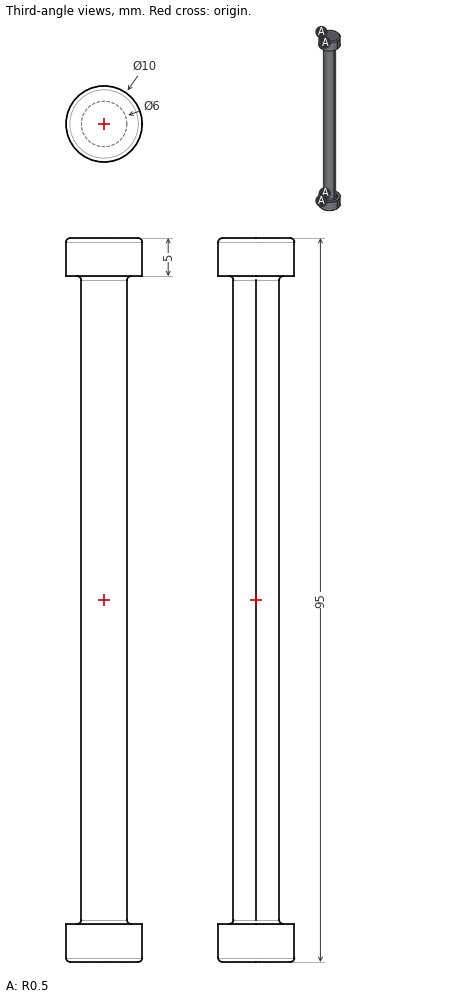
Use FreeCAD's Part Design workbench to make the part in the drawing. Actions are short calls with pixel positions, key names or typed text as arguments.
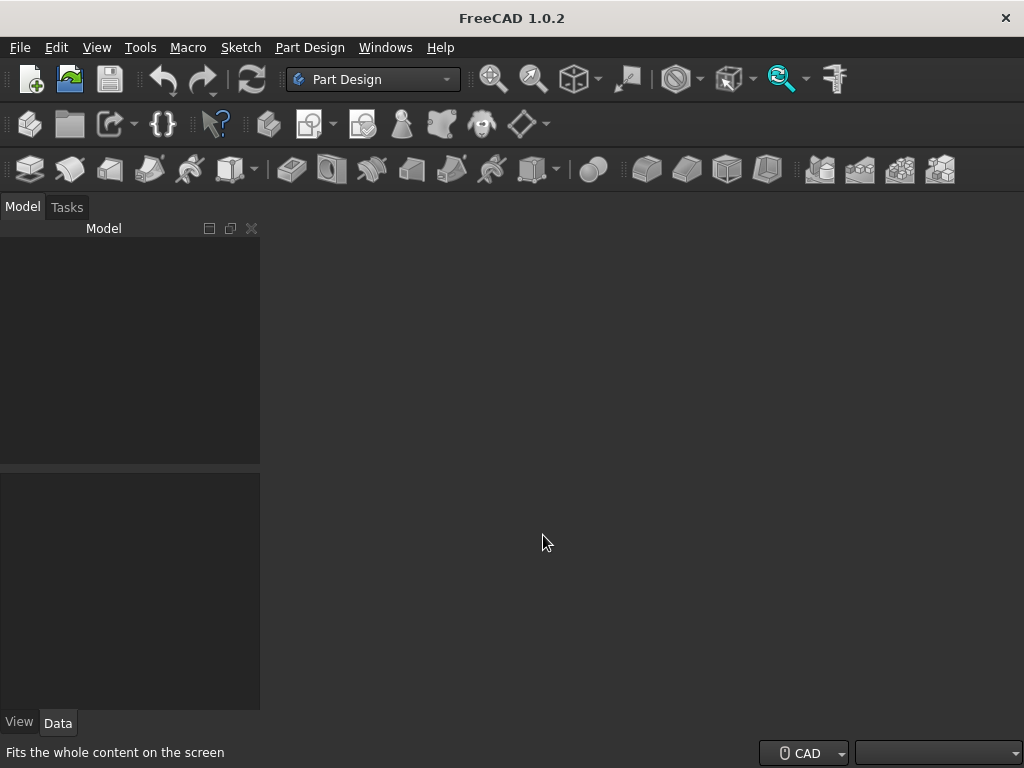
click(30, 80)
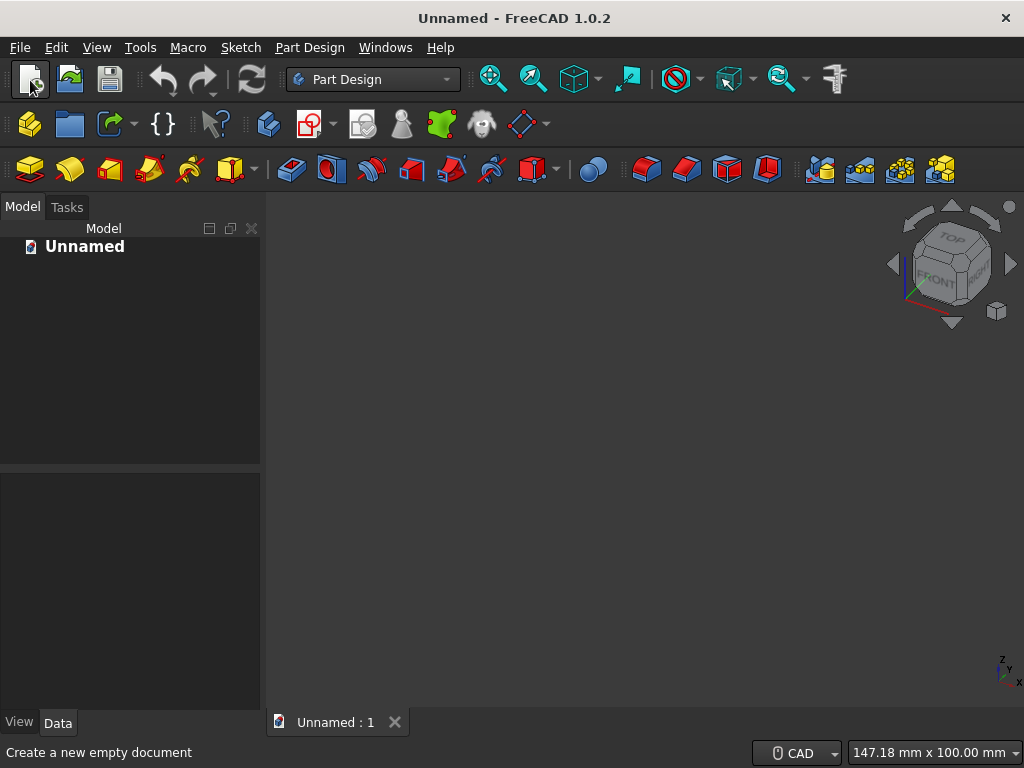
click(310, 124)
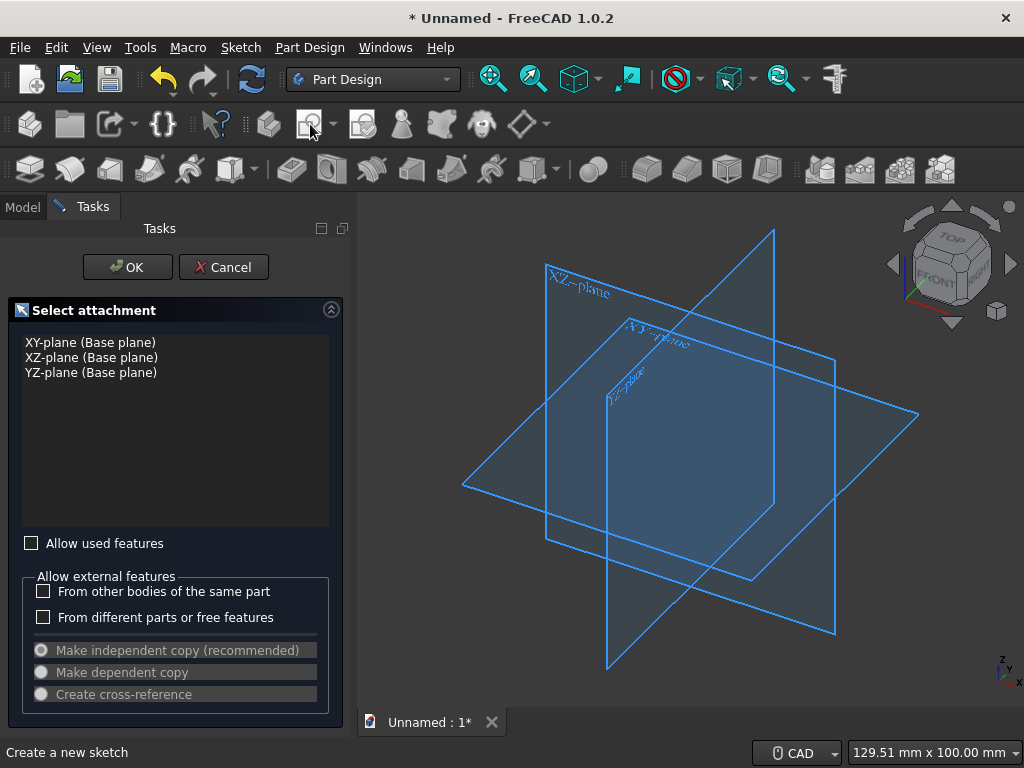
click(82, 342)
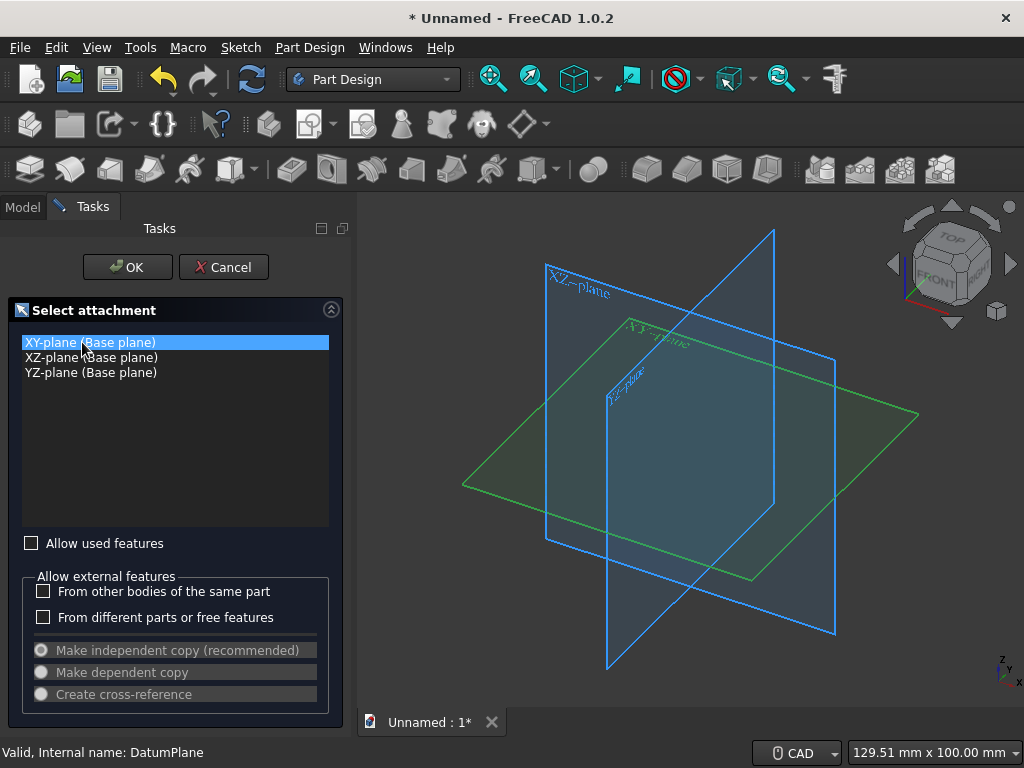
click(128, 267)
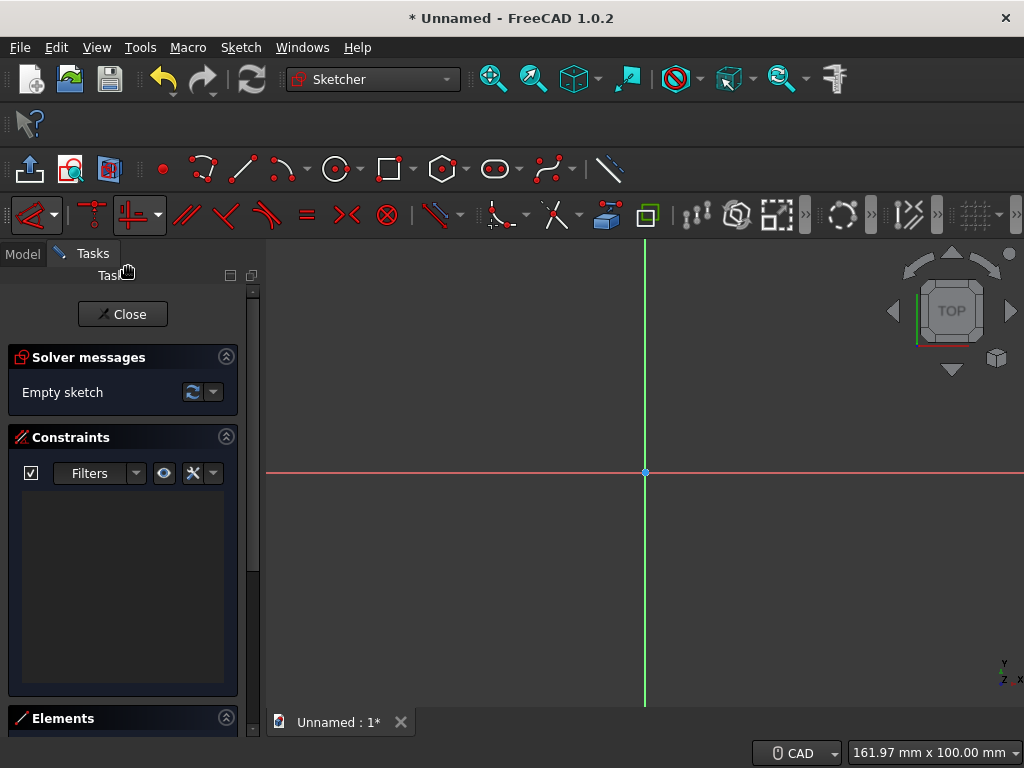
scroll(652, 473, up, 12)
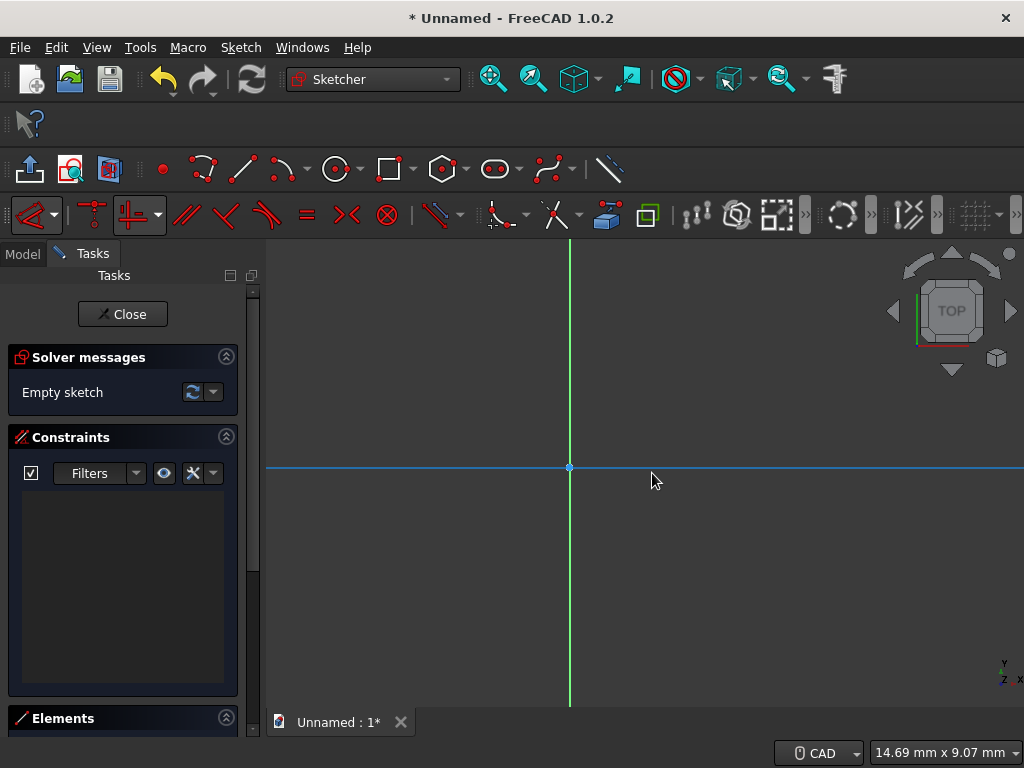
click(336, 170)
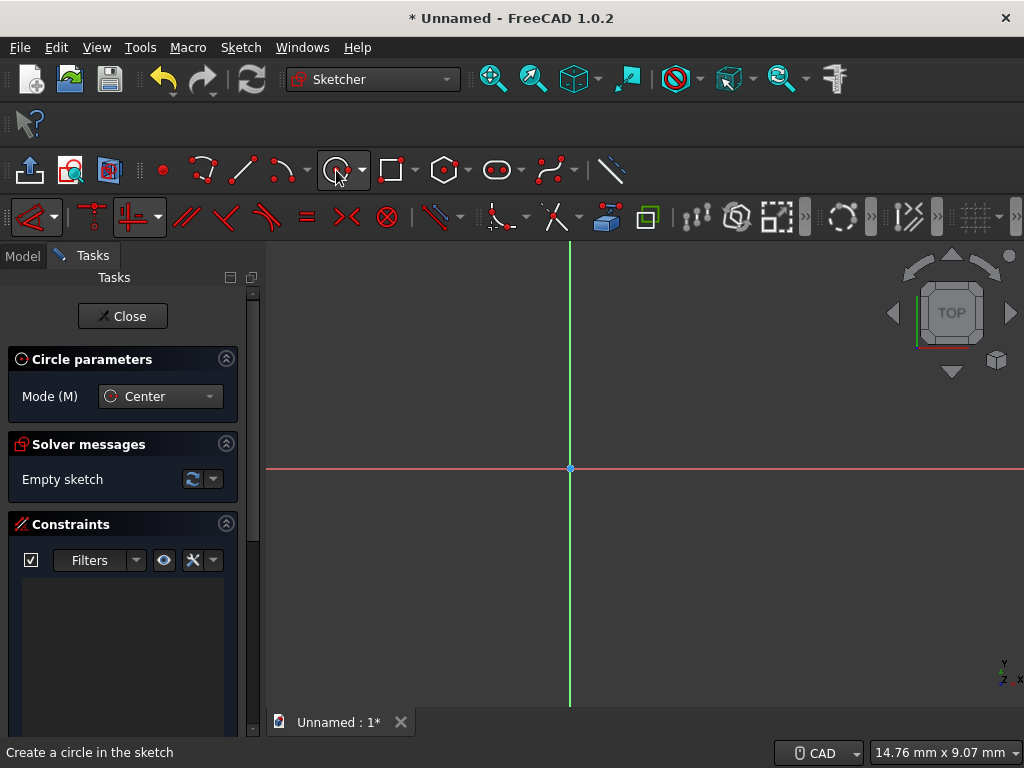
click(570, 469)
move(679, 360)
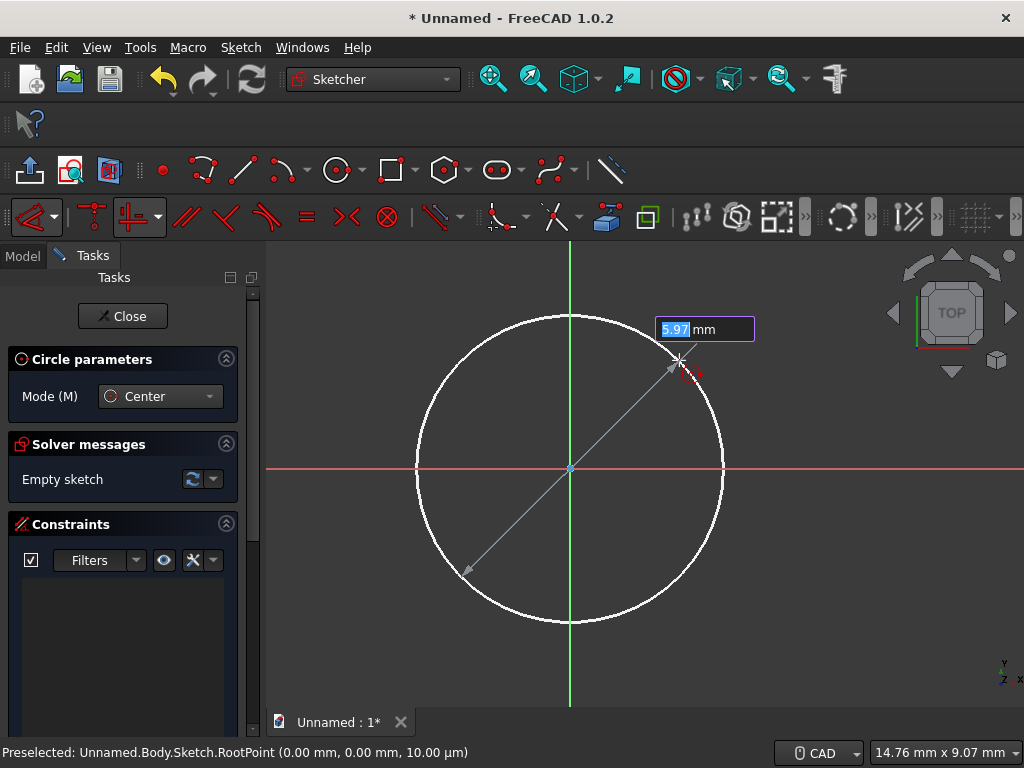
text(6)
key(Return)
key(Escape)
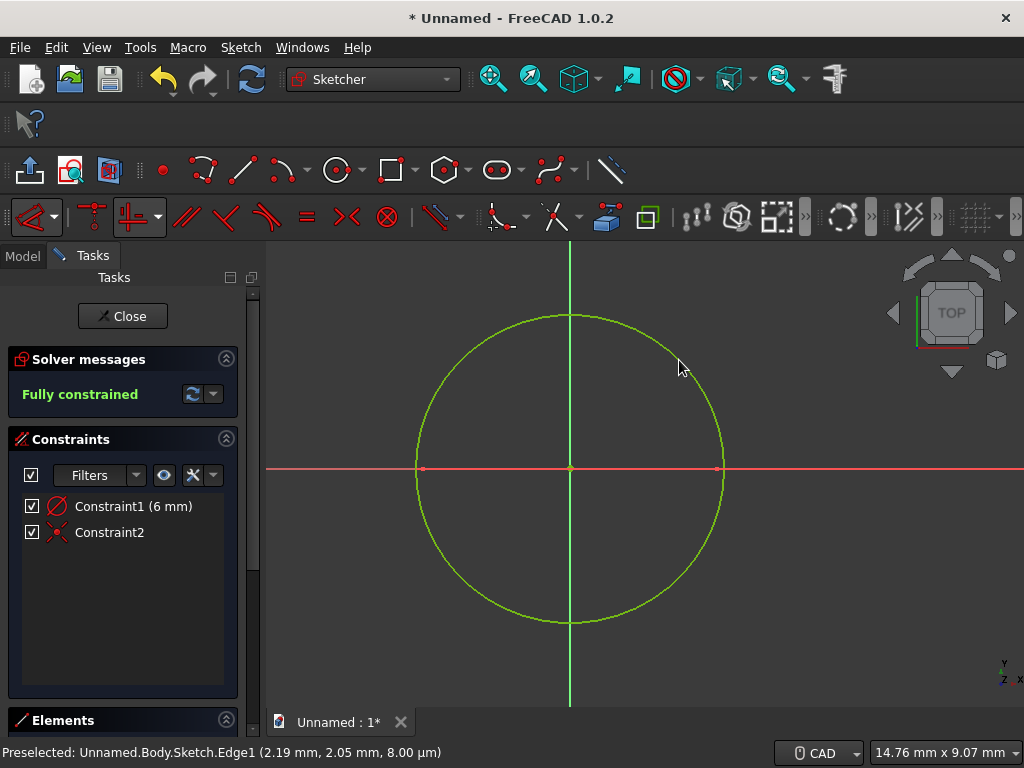
click(123, 316)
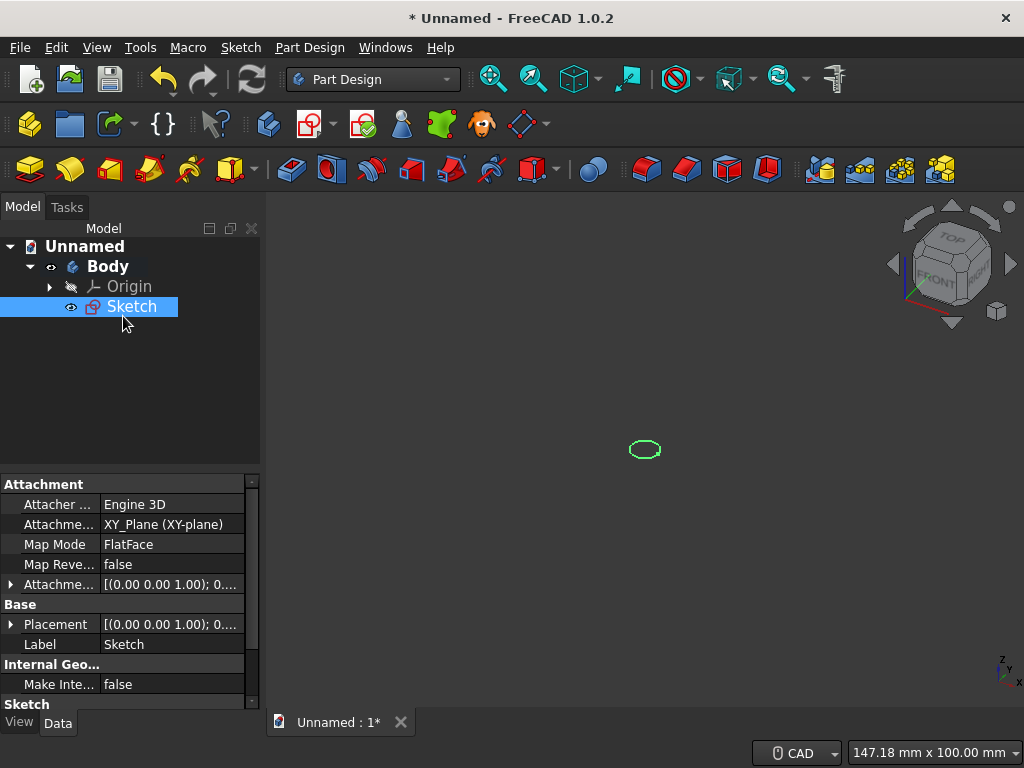
click(30, 170)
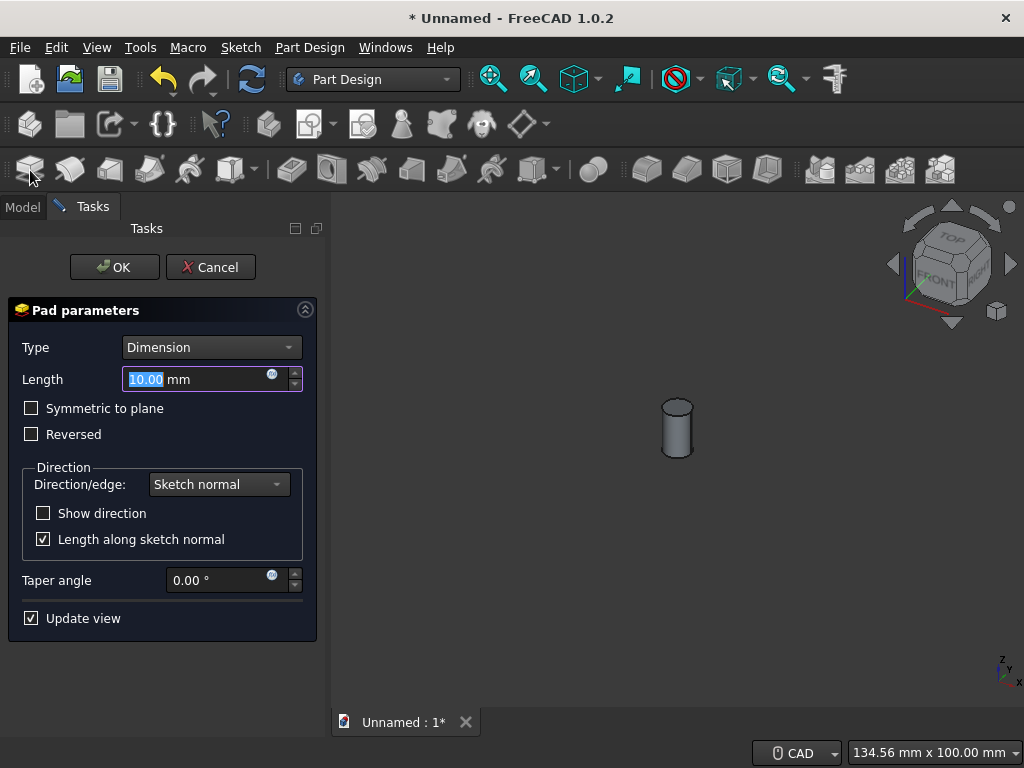
text(95)
key(Tab)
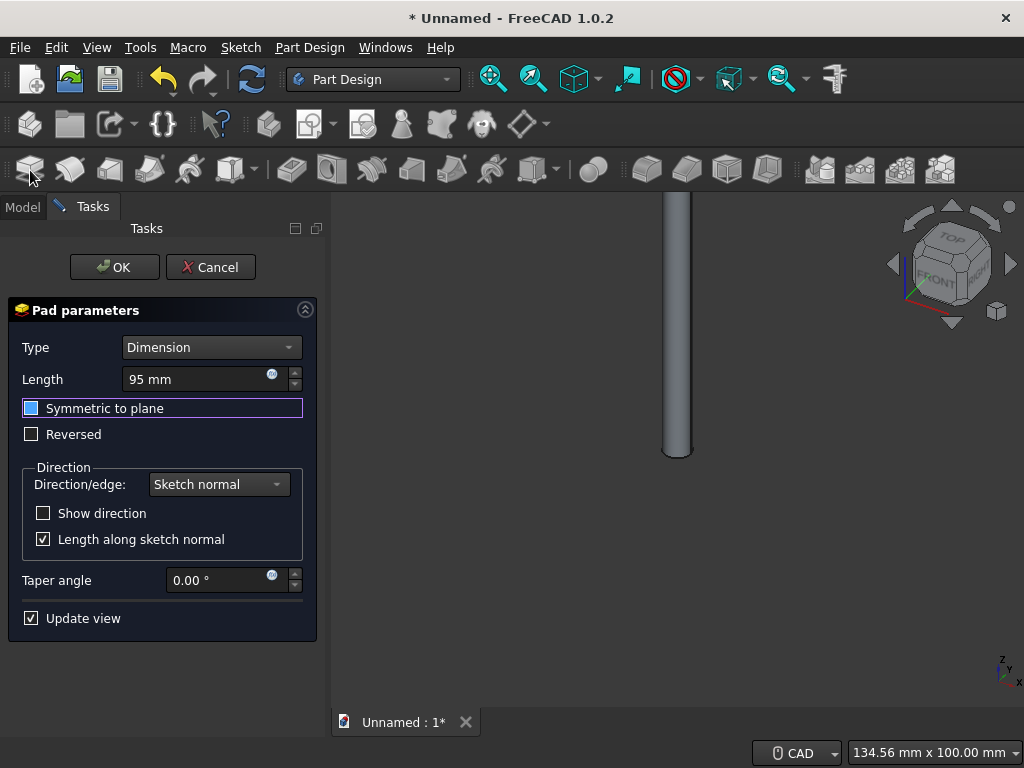
click(30, 408)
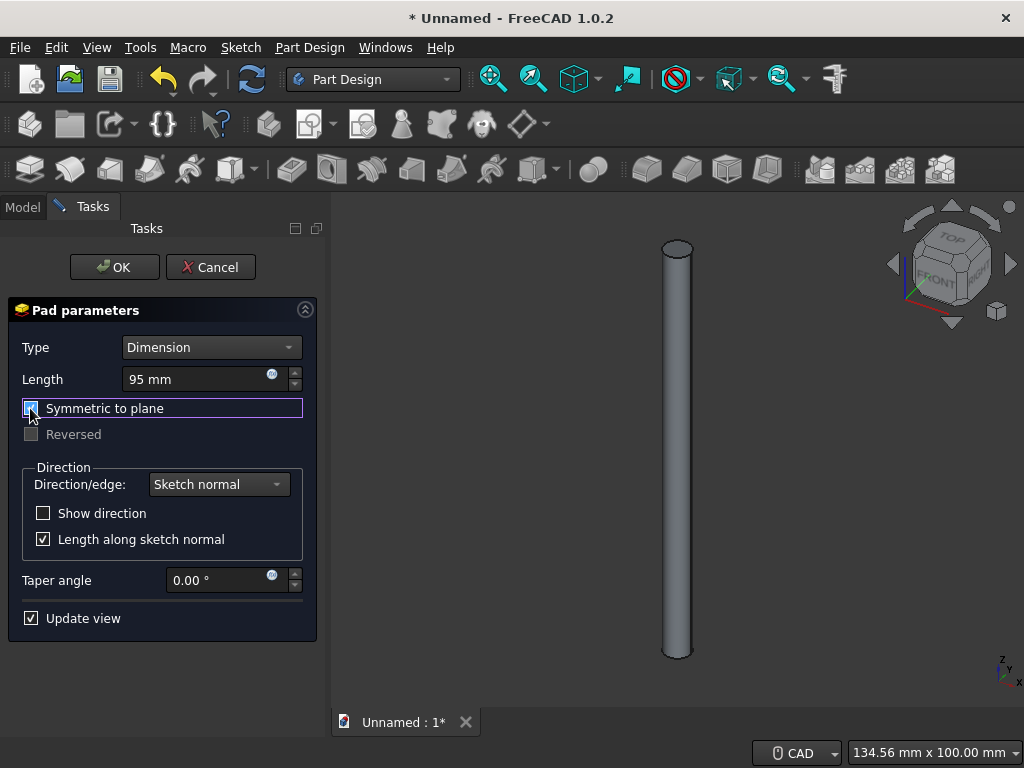
click(115, 267)